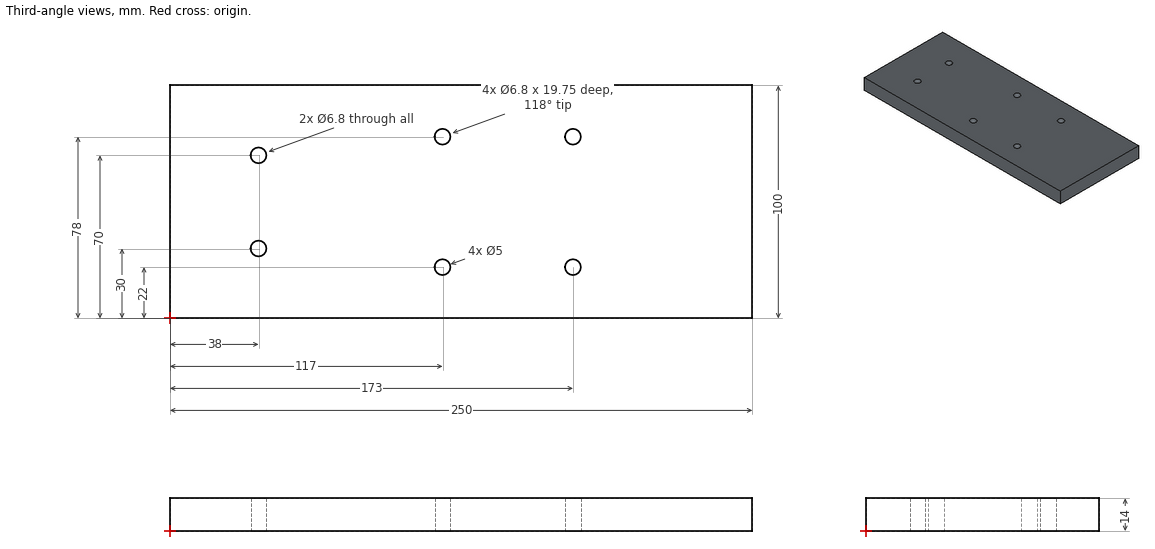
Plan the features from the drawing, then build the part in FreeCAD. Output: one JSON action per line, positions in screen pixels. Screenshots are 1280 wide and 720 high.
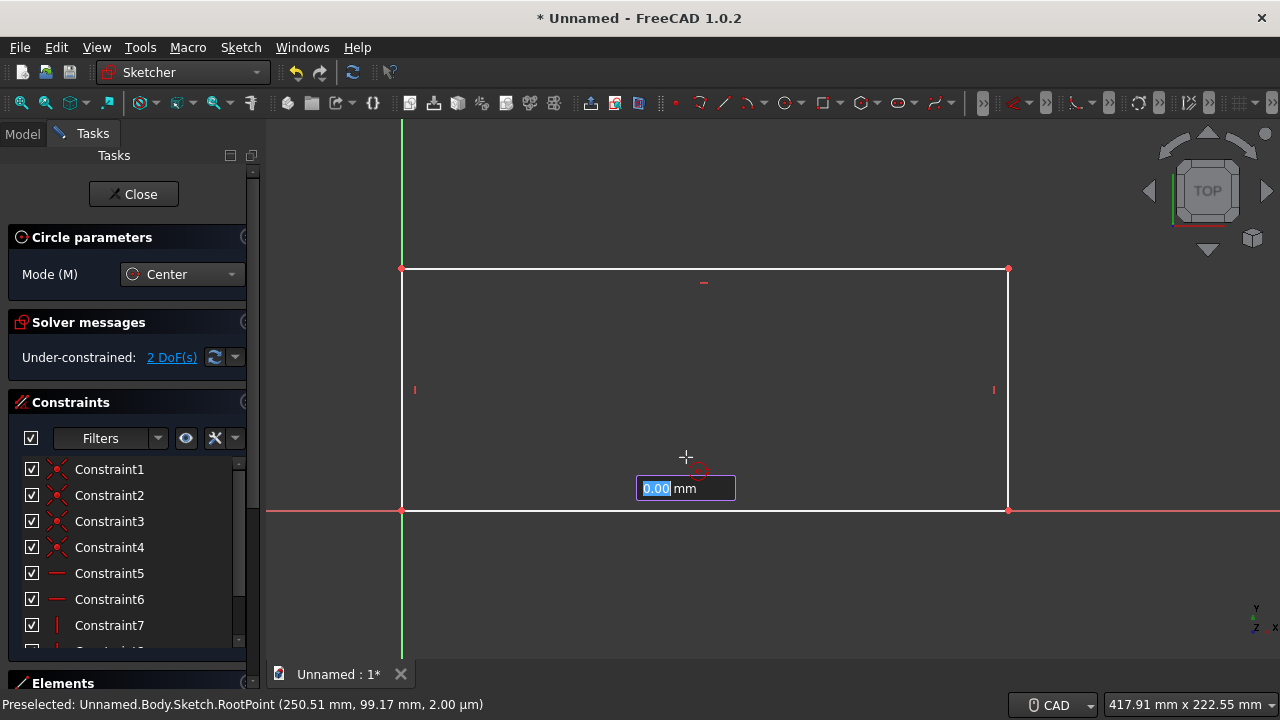
{"action": "scroll", "coordinate": [690, 453], "scroll_direction": "up", "scroll_amount": 5}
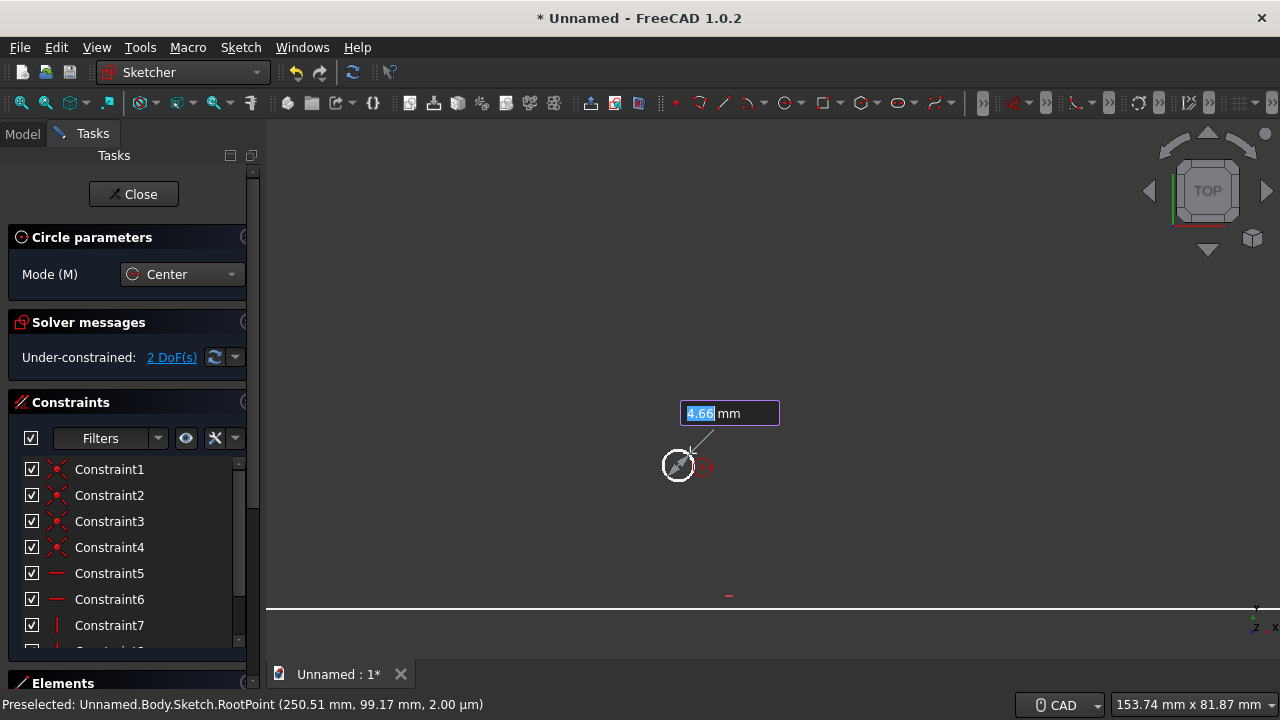
{"action": "left_click", "coordinate": [689, 452]}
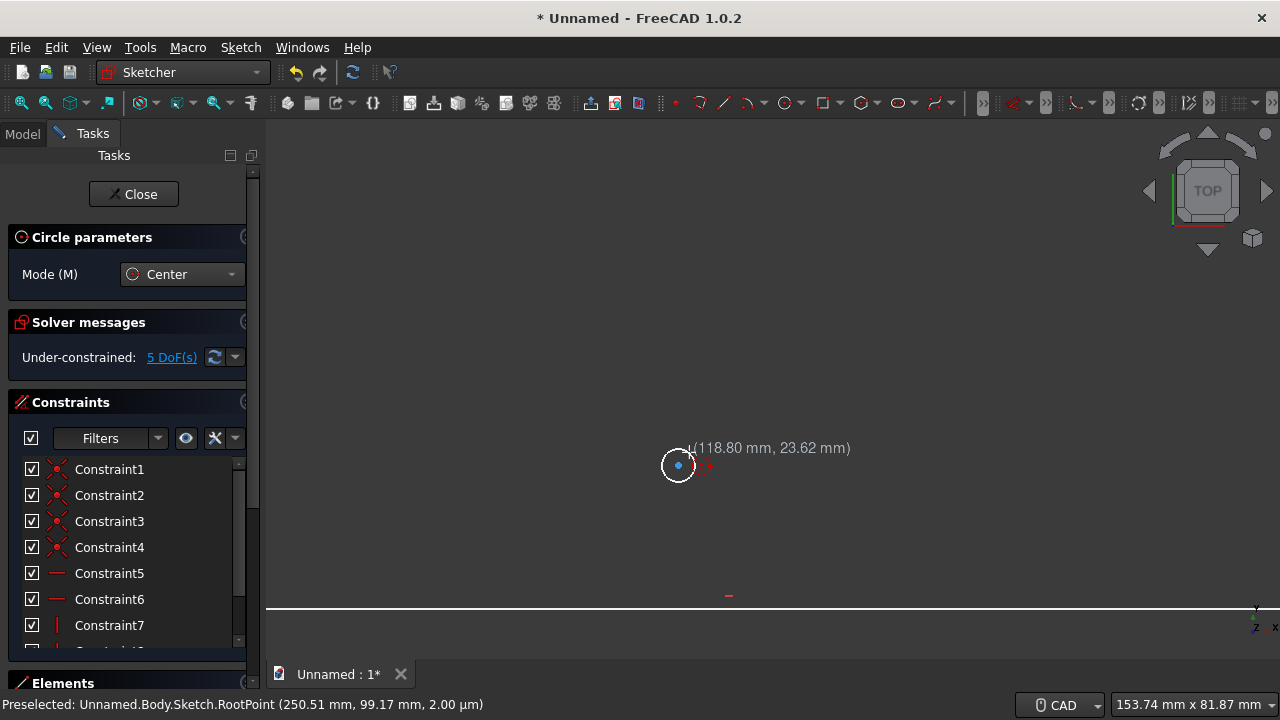
{"action": "scroll", "coordinate": [1046, 464], "scroll_direction": "up", "scroll_amount": 2}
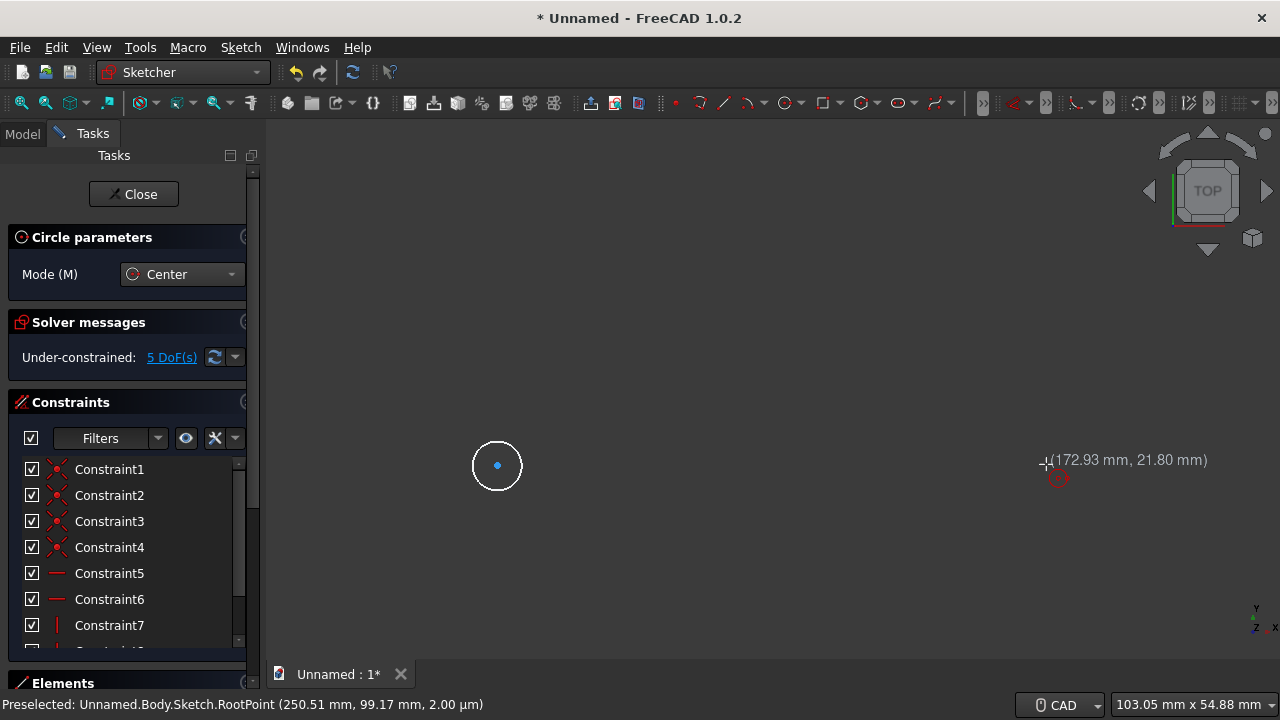
{"action": "scroll", "coordinate": [747, 455], "scroll_direction": "down", "scroll_amount": 7}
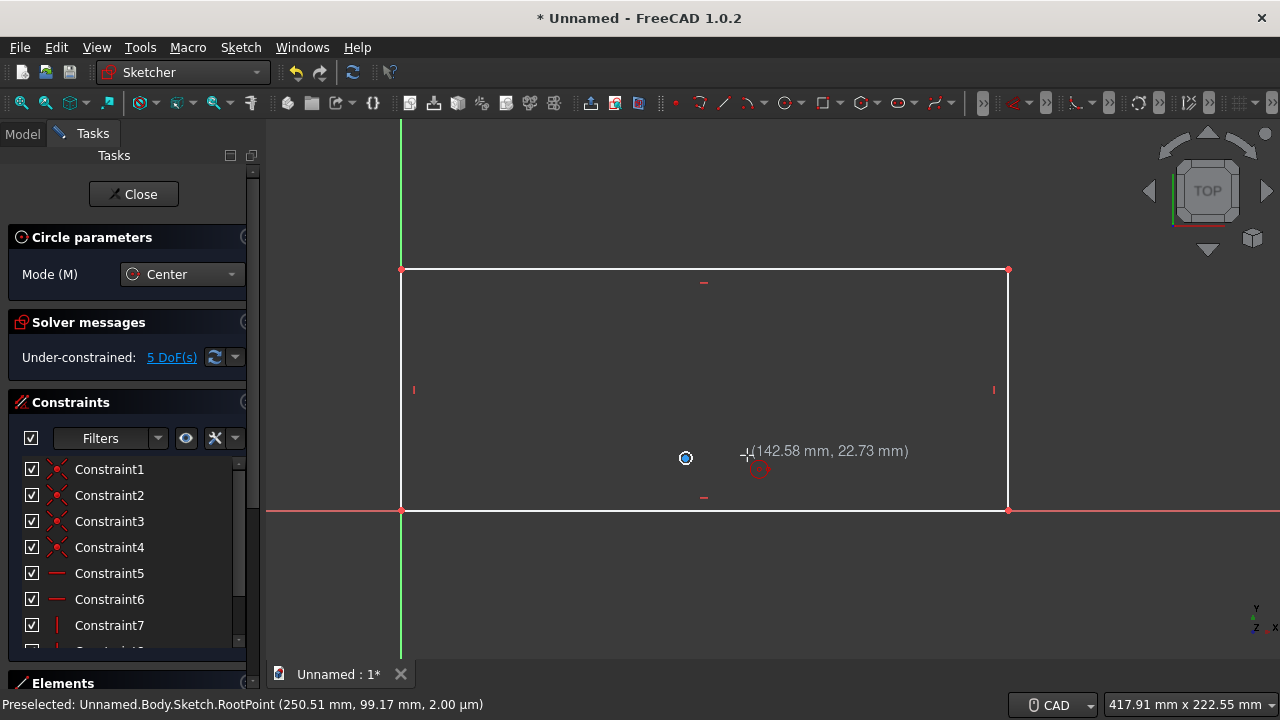
{"action": "left_click", "coordinate": [821, 457]}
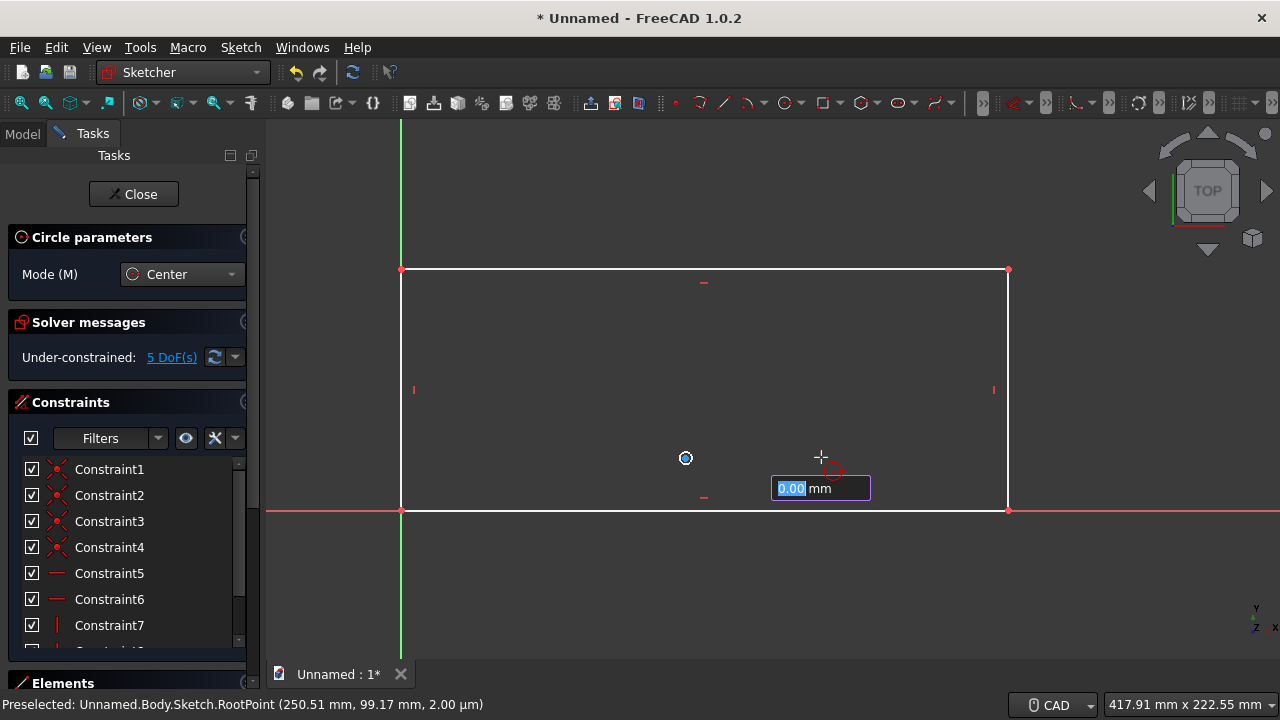
{"action": "scroll", "coordinate": [825, 453], "scroll_direction": "up", "scroll_amount": 5}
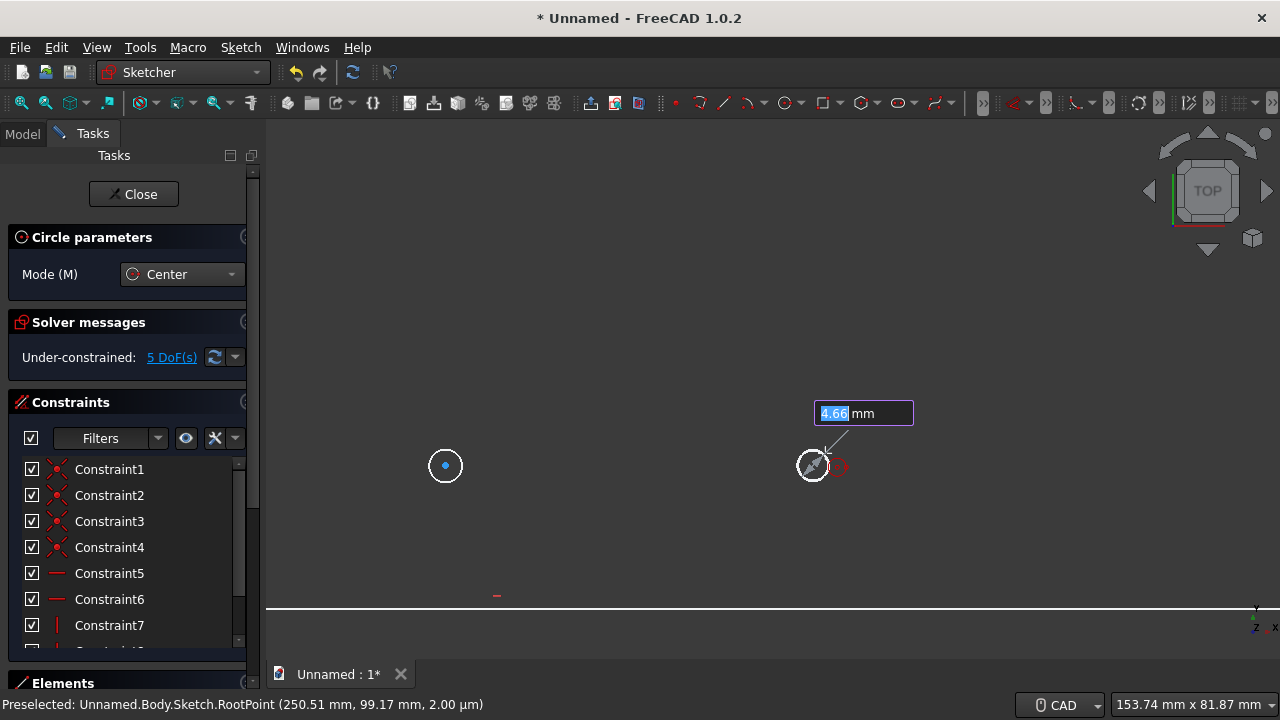
{"action": "left_click", "coordinate": [825, 452]}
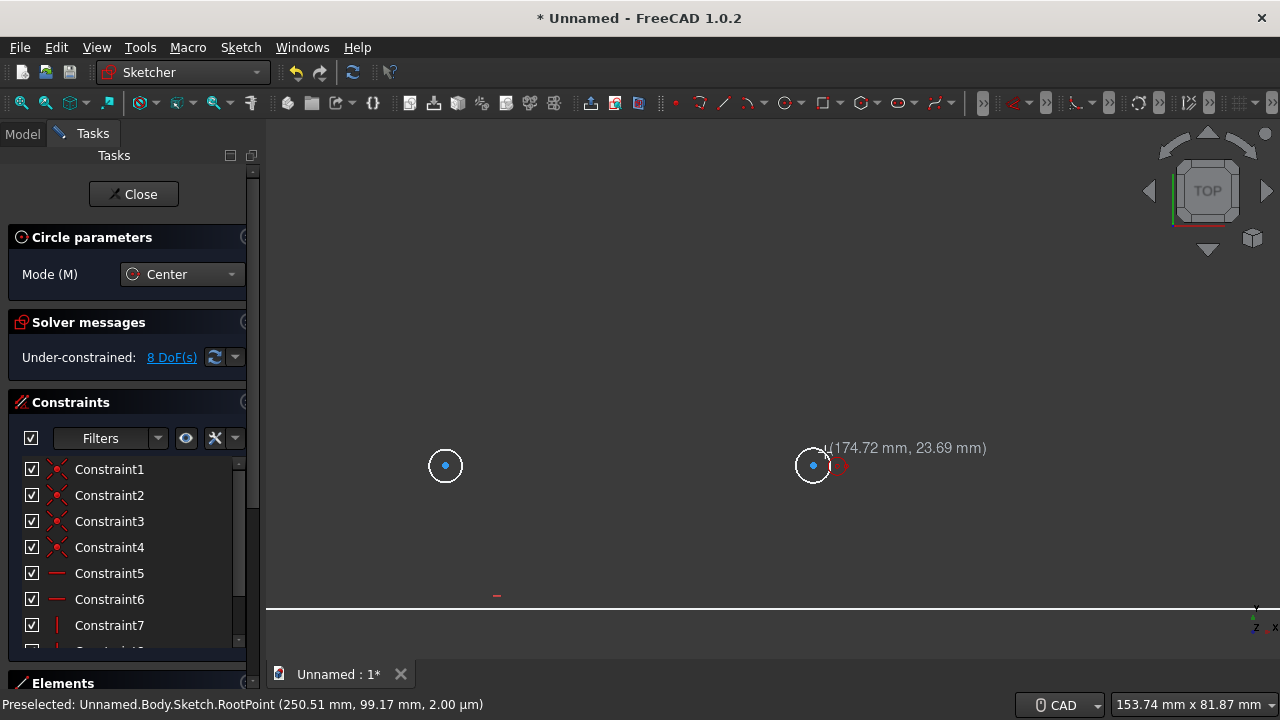
{"action": "scroll", "coordinate": [825, 453], "scroll_direction": "down", "scroll_amount": 5}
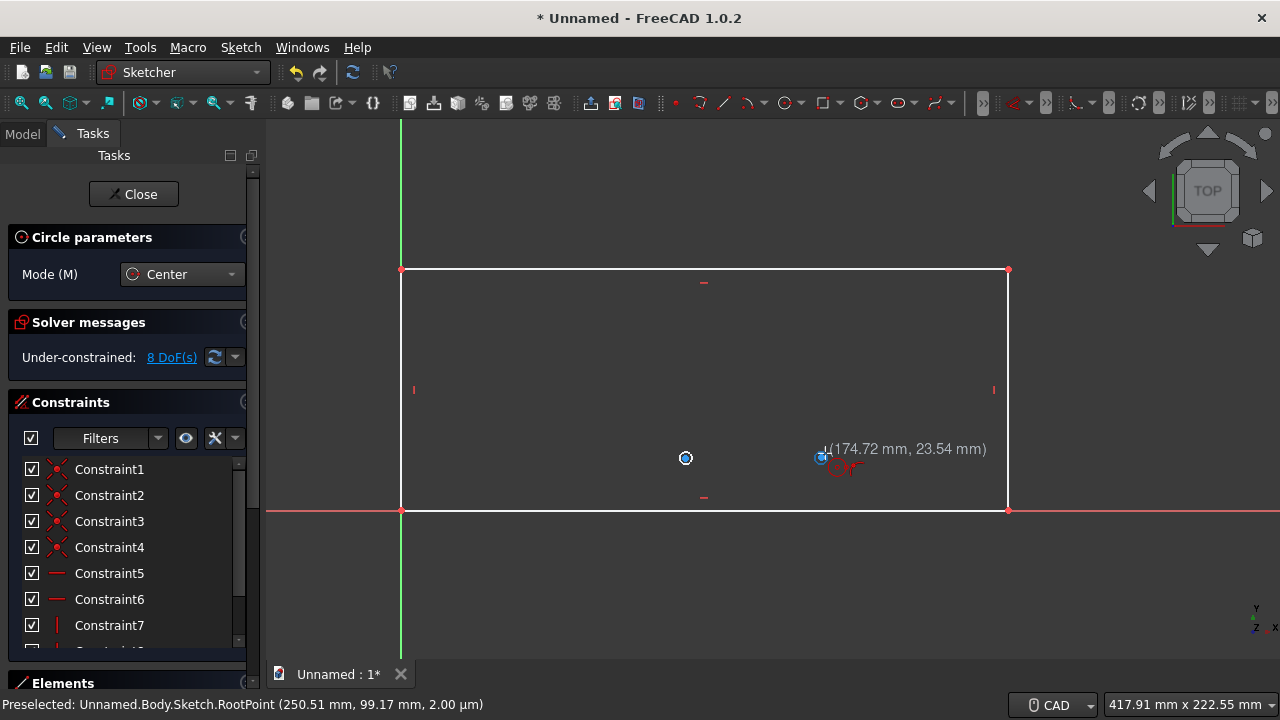
{"action": "scroll", "coordinate": [685, 322], "scroll_direction": "up", "scroll_amount": 7}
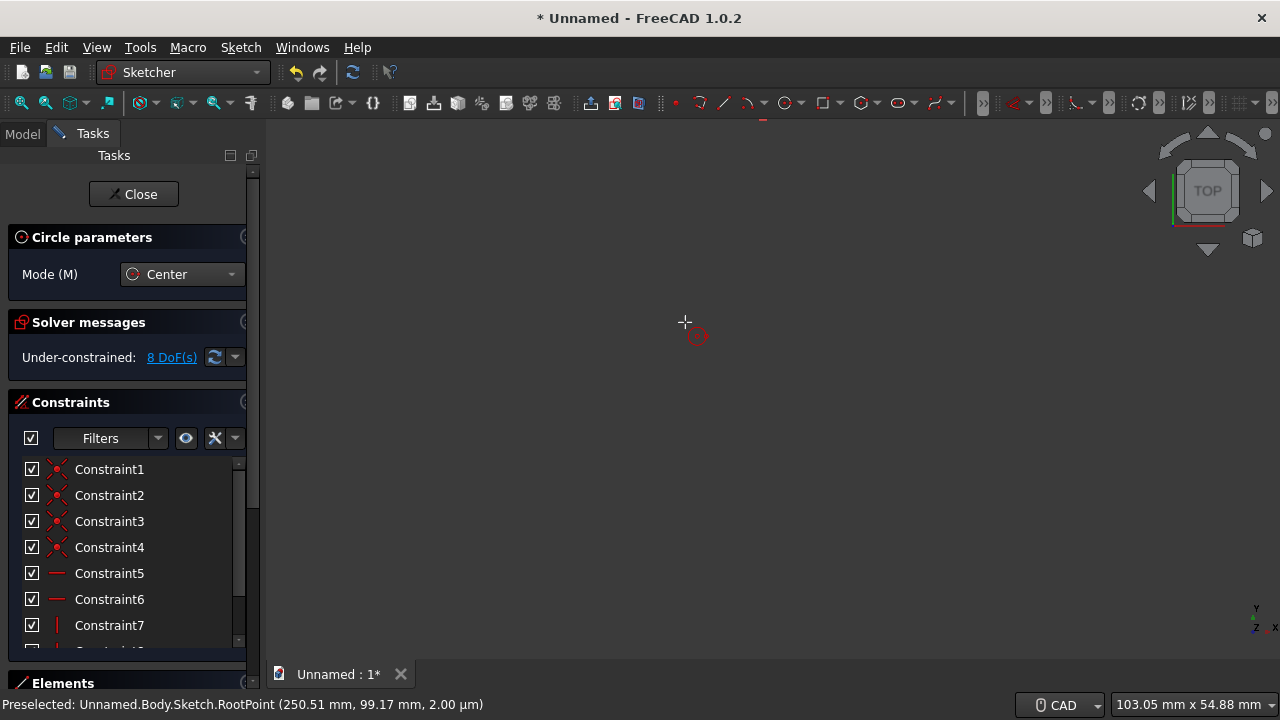
{"action": "scroll", "coordinate": [685, 322], "scroll_direction": "down", "scroll_amount": 7}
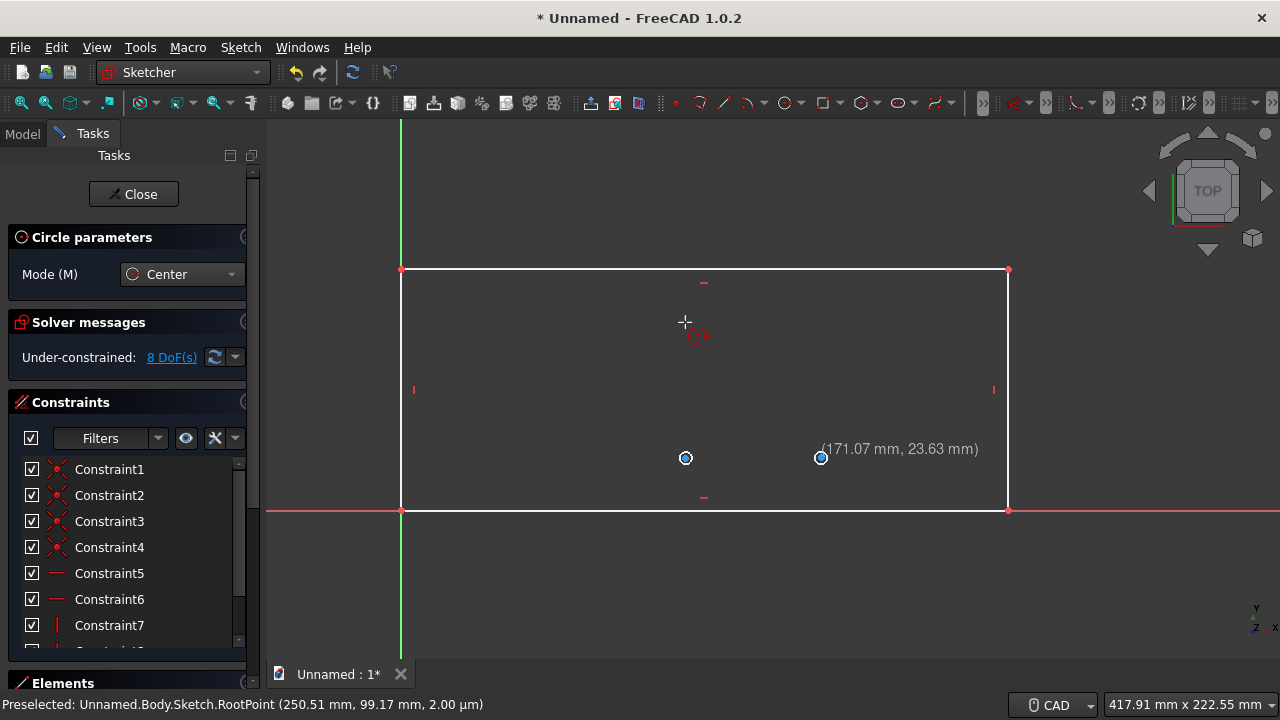
{"action": "left_click", "coordinate": [685, 322]}